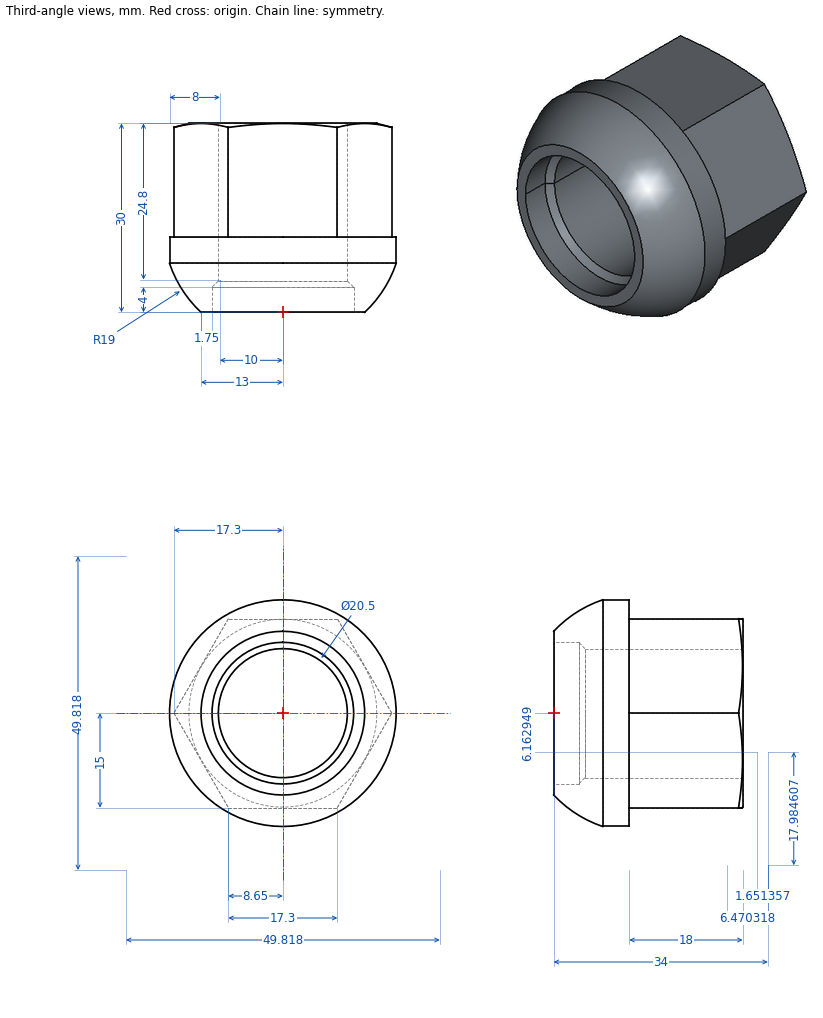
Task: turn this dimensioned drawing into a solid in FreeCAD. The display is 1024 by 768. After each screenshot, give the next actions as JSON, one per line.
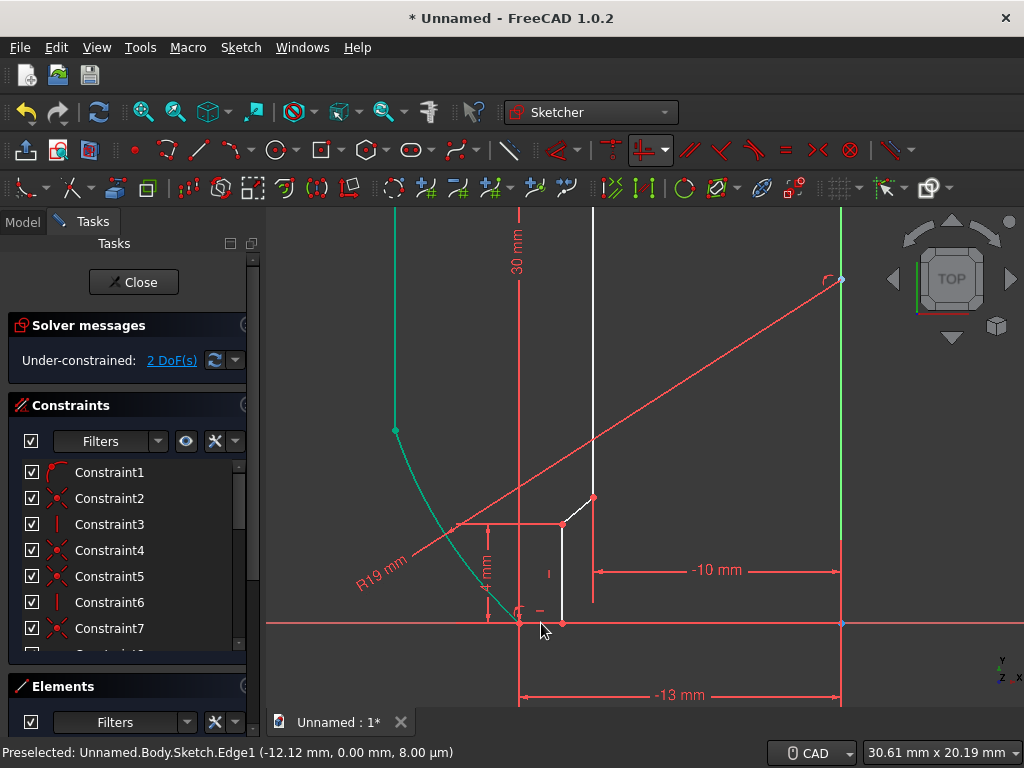
{"action": "left_click", "coordinate": [580, 150]}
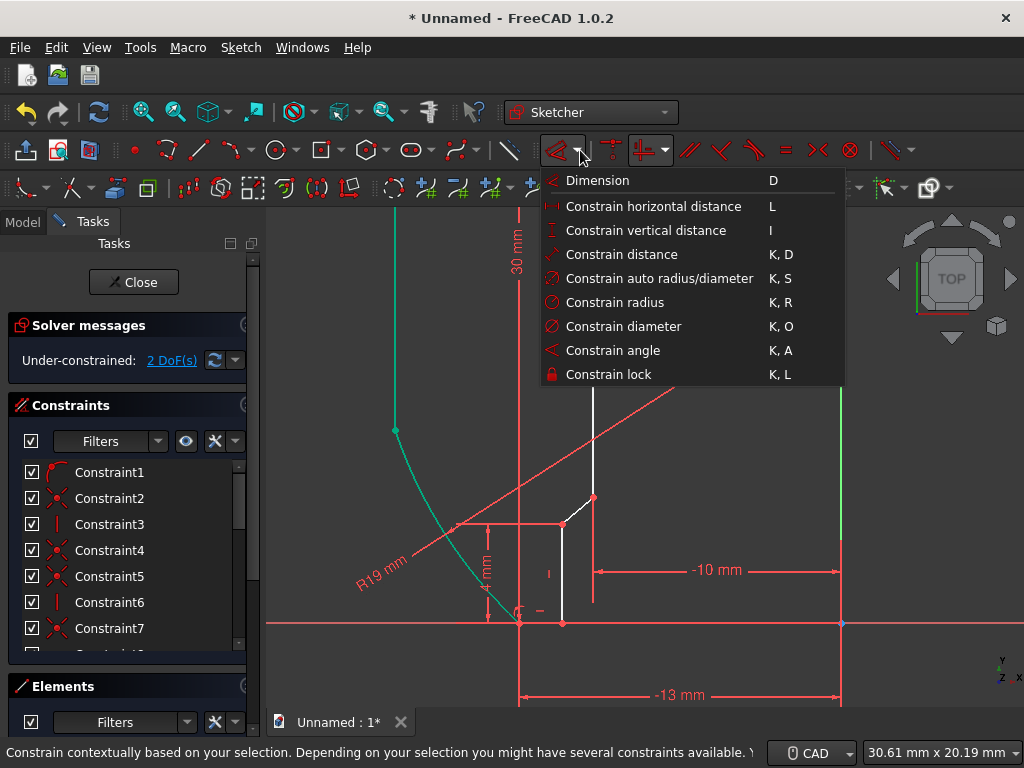
{"action": "left_click", "coordinate": [693, 206]}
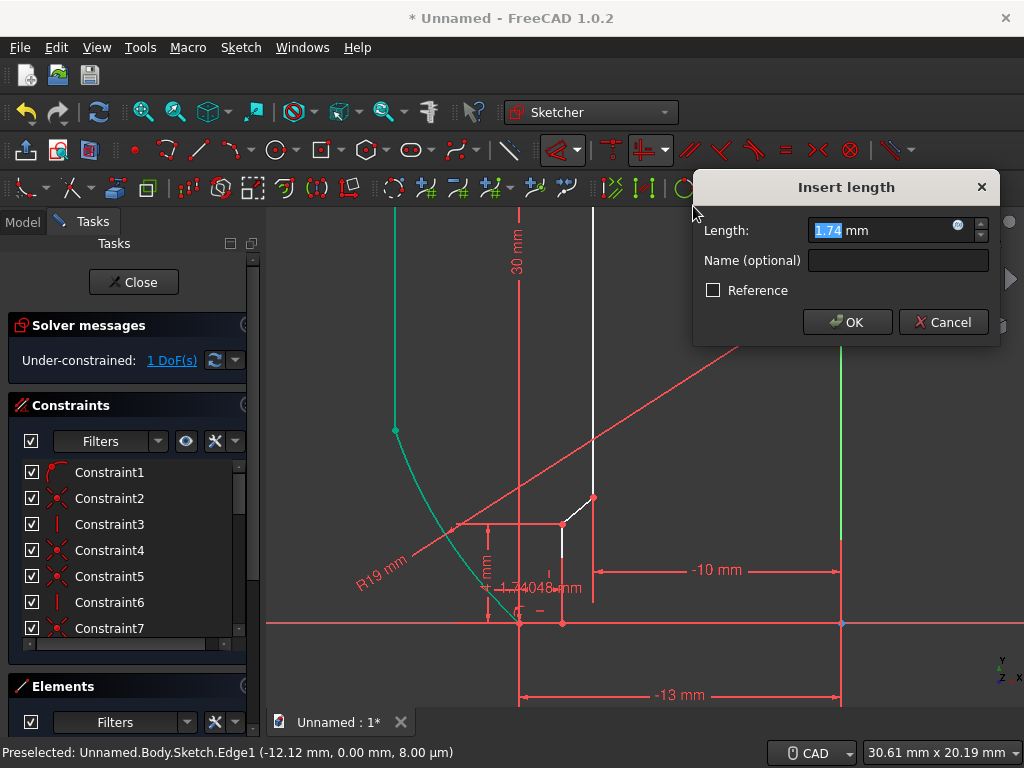
{"action": "type", "text": "1.75"}
{"action": "key", "text": "Return"}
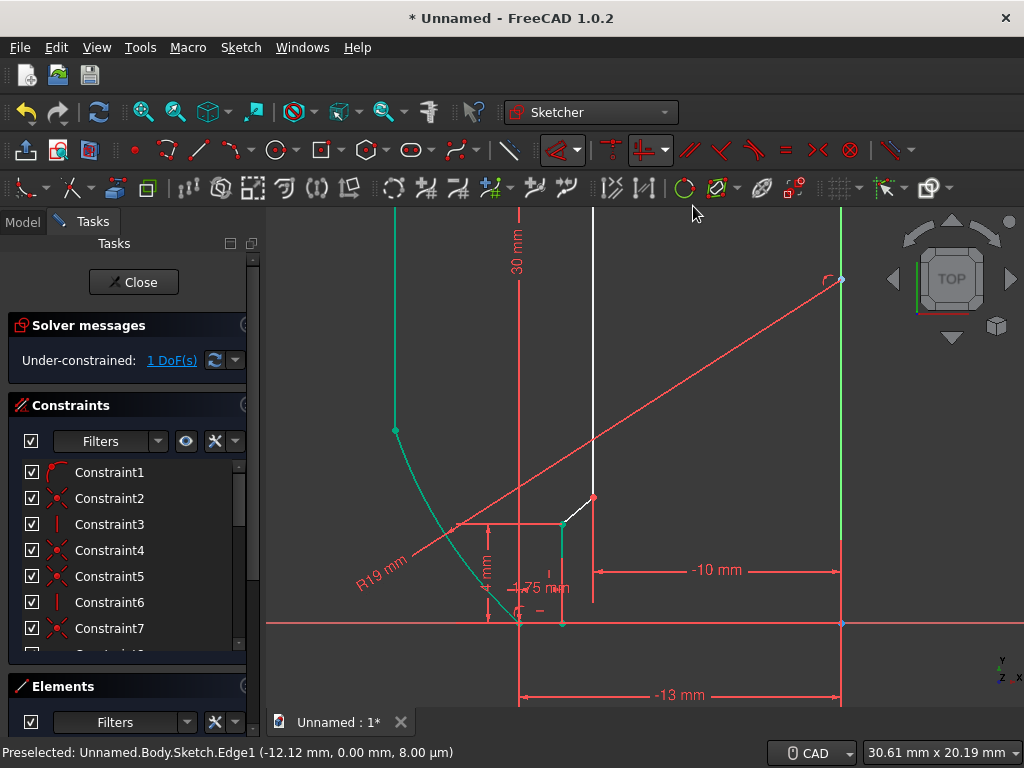
{"action": "left_click", "coordinate": [593, 312]}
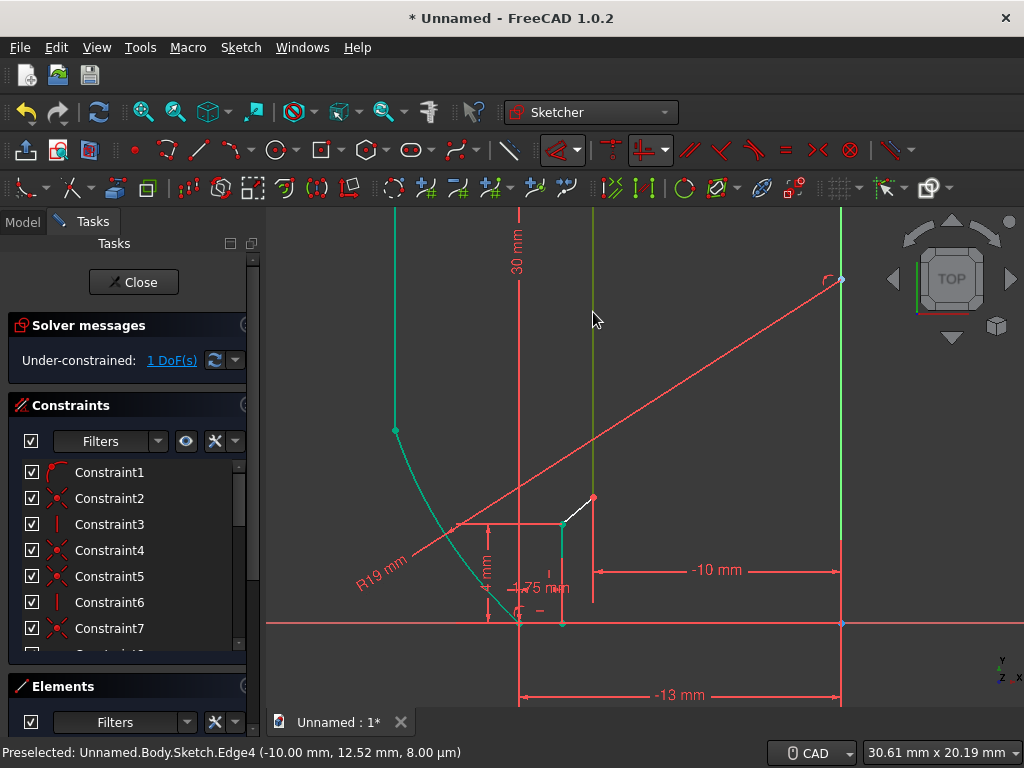
{"action": "key", "text": "i"}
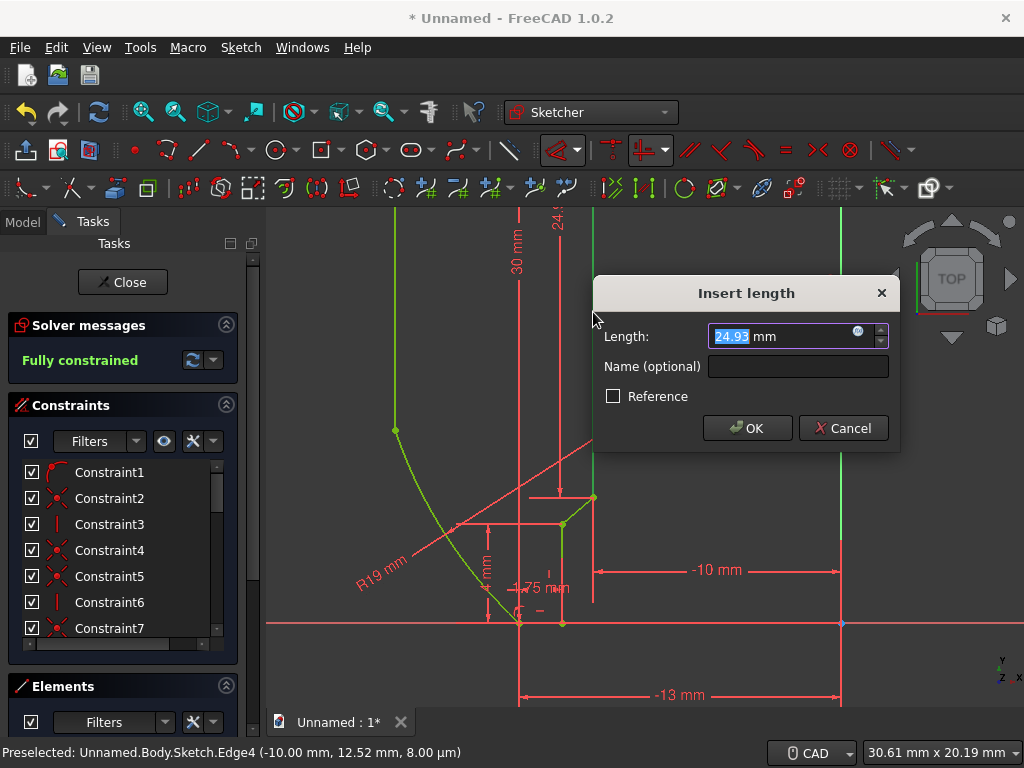
{"action": "type", "text": "24.8"}
{"action": "key", "text": "Return"}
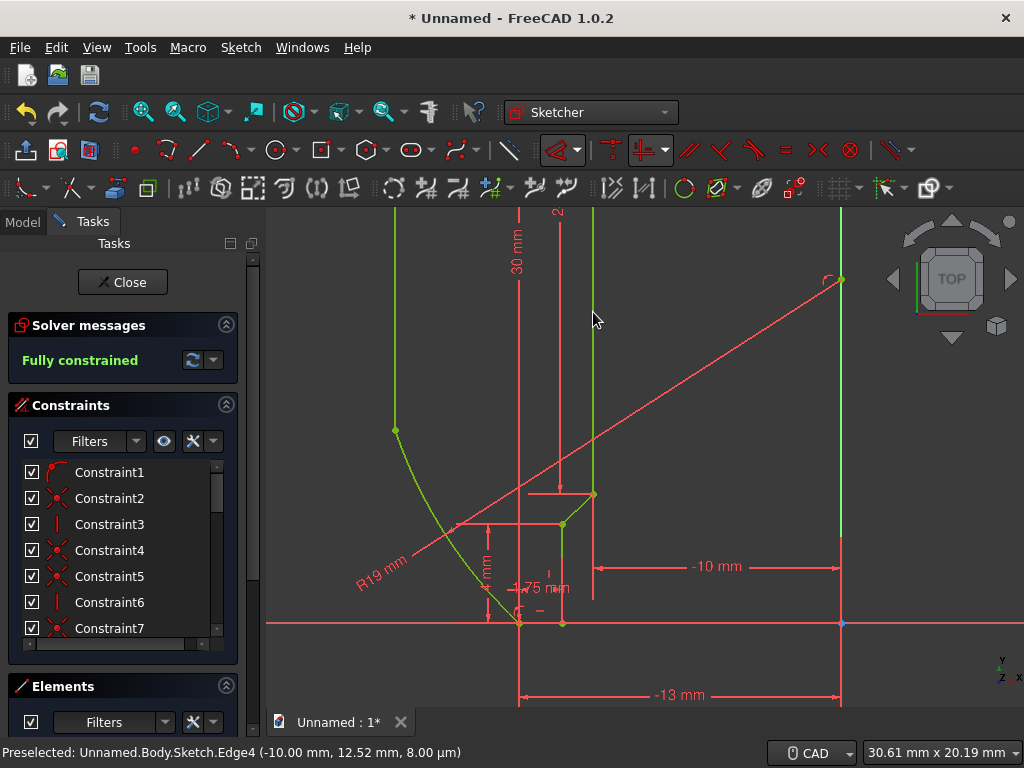
{"action": "left_click", "coordinate": [123, 282]}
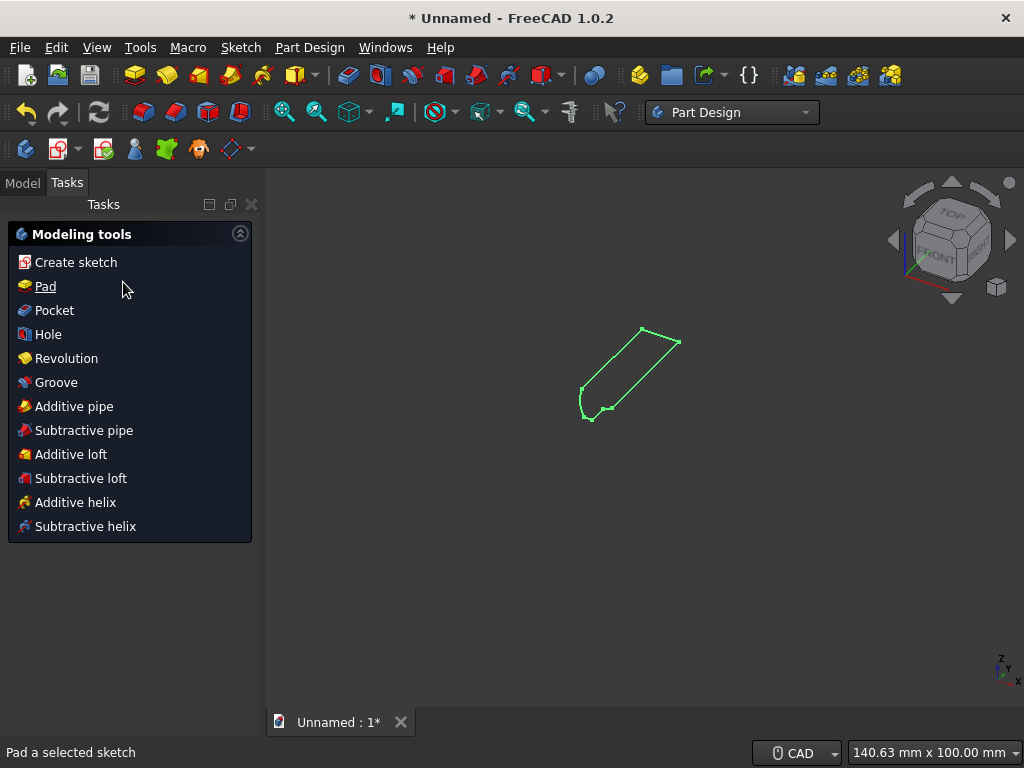
{"action": "left_click", "coordinate": [168, 76]}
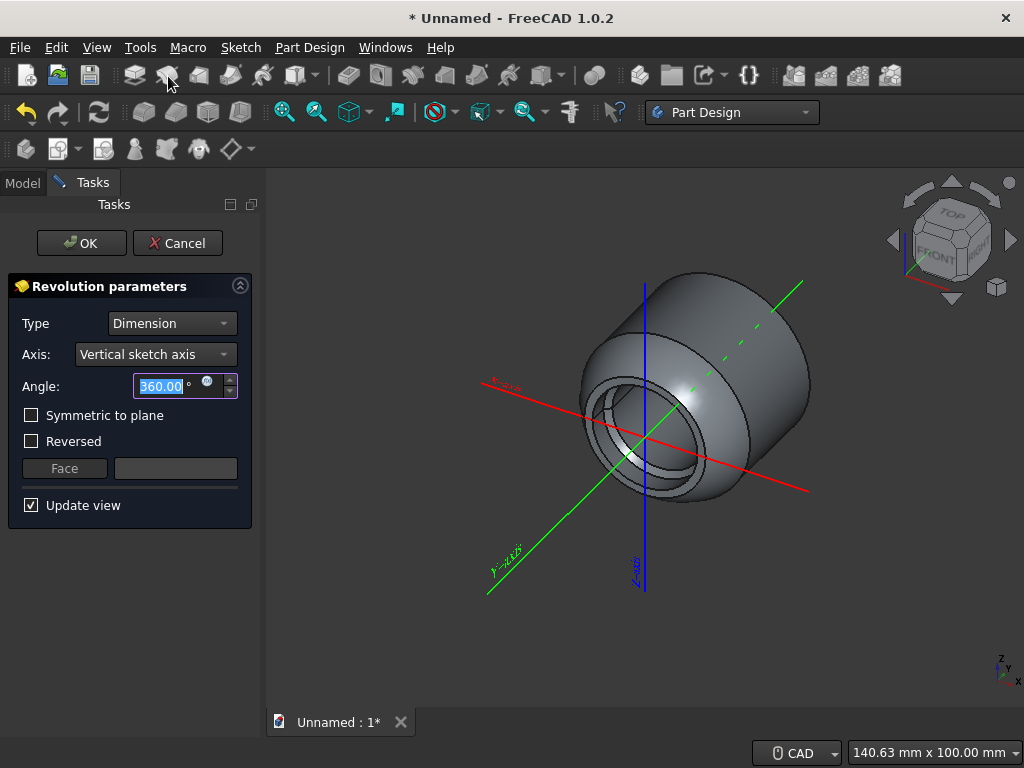
{"action": "left_click", "coordinate": [82, 243]}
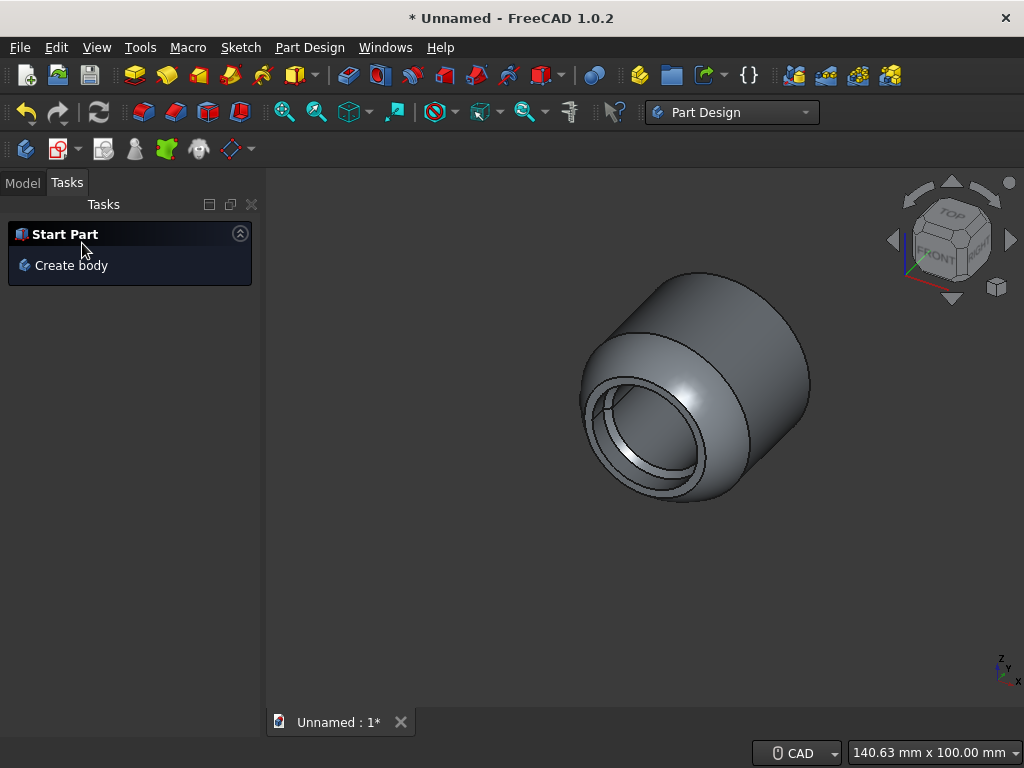
{"action": "key", "text": "4"}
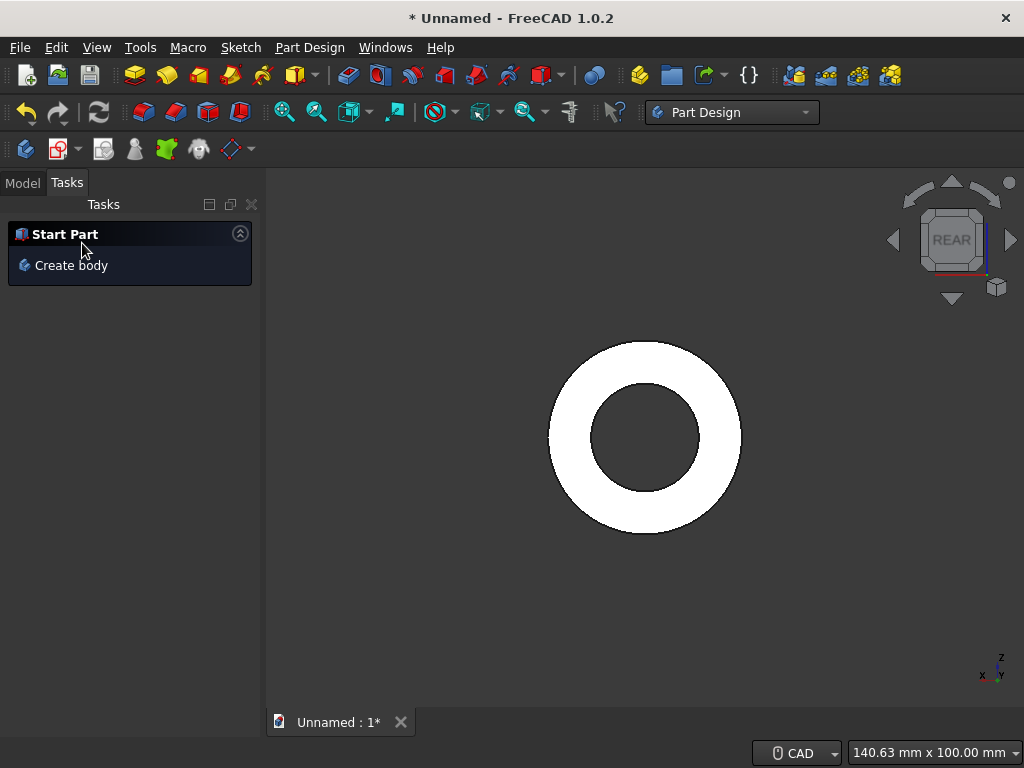
{"action": "key", "text": "v f"}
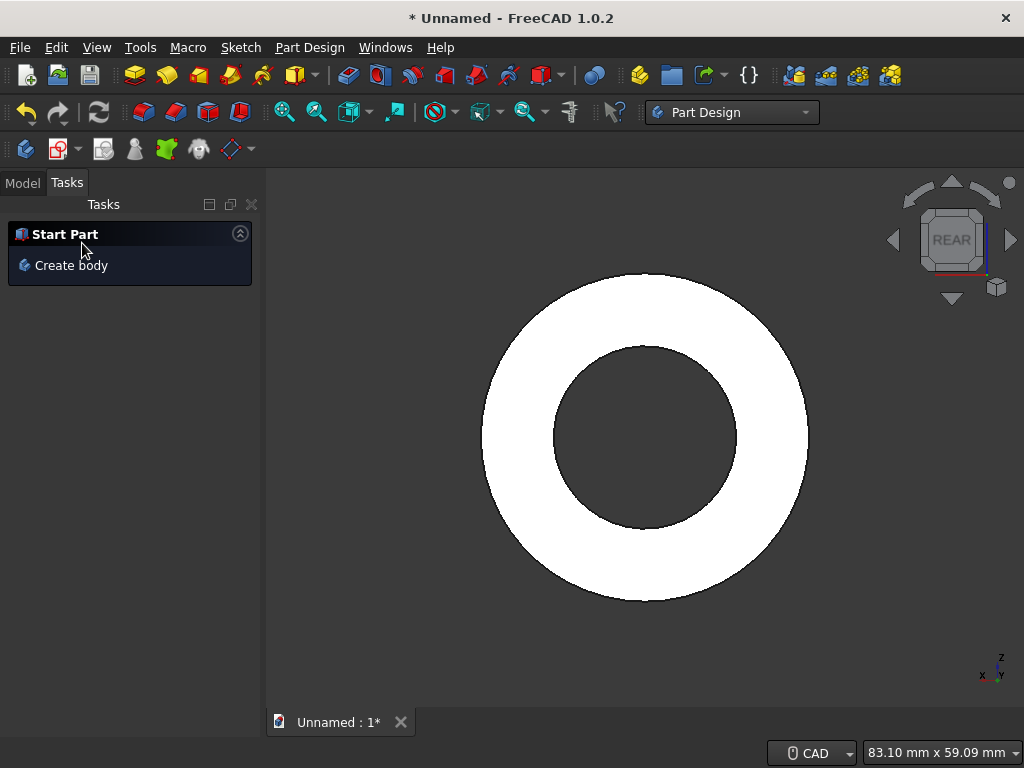
{"action": "left_click", "coordinate": [551, 530]}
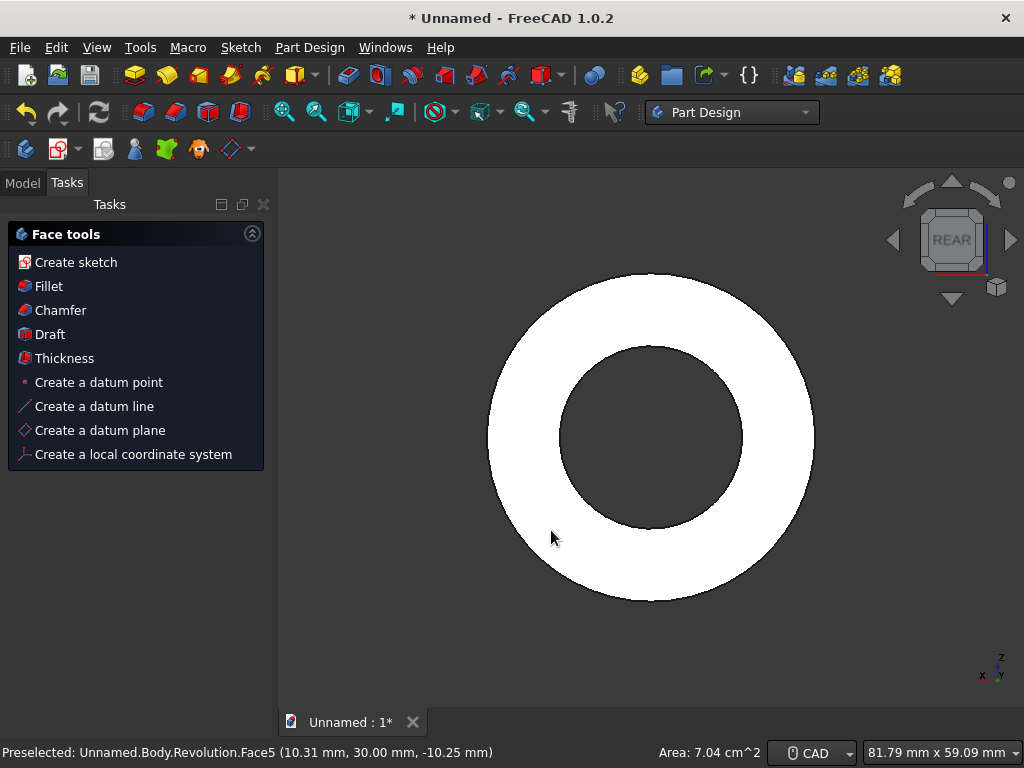
{"action": "left_click", "coordinate": [58, 150]}